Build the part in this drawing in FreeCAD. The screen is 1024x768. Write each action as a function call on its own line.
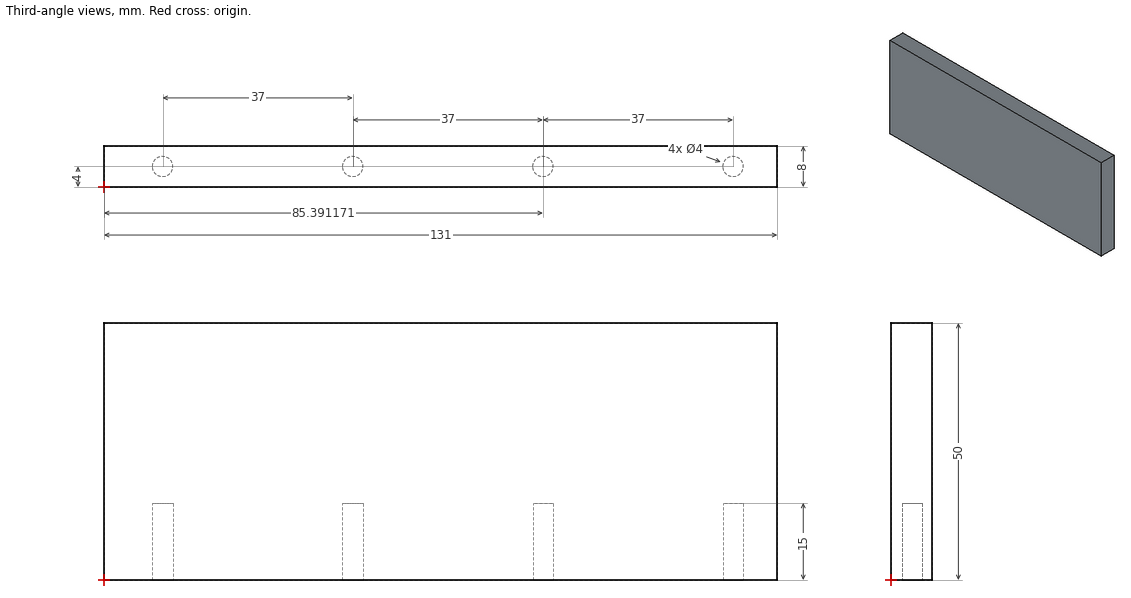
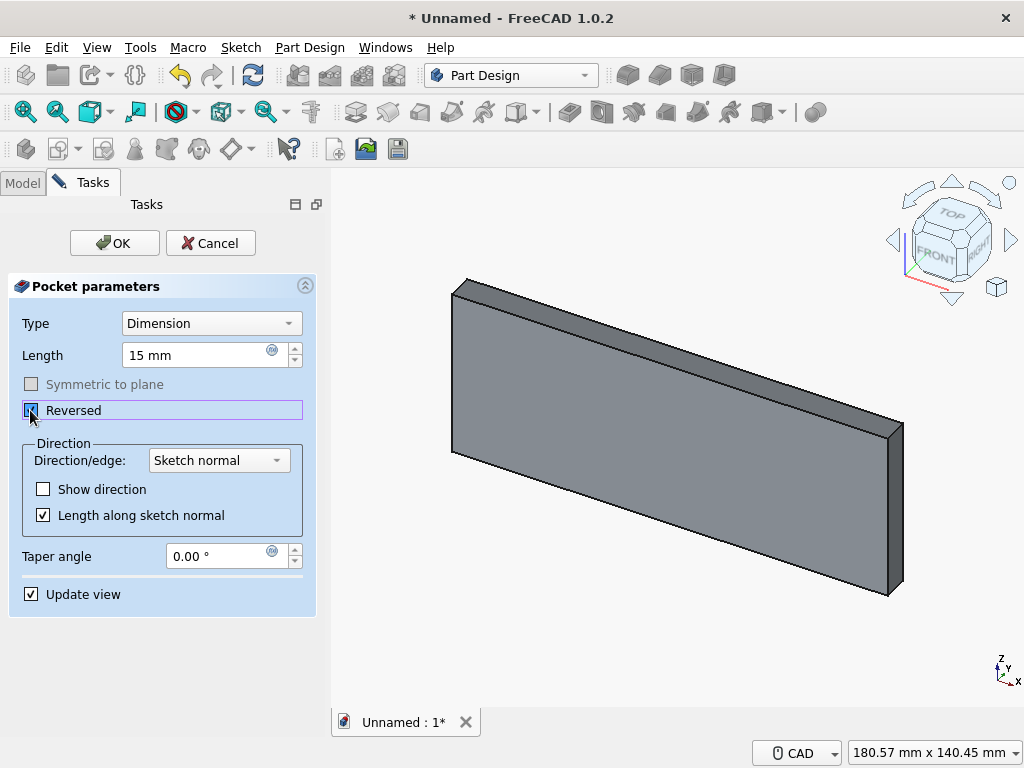
click(115, 243)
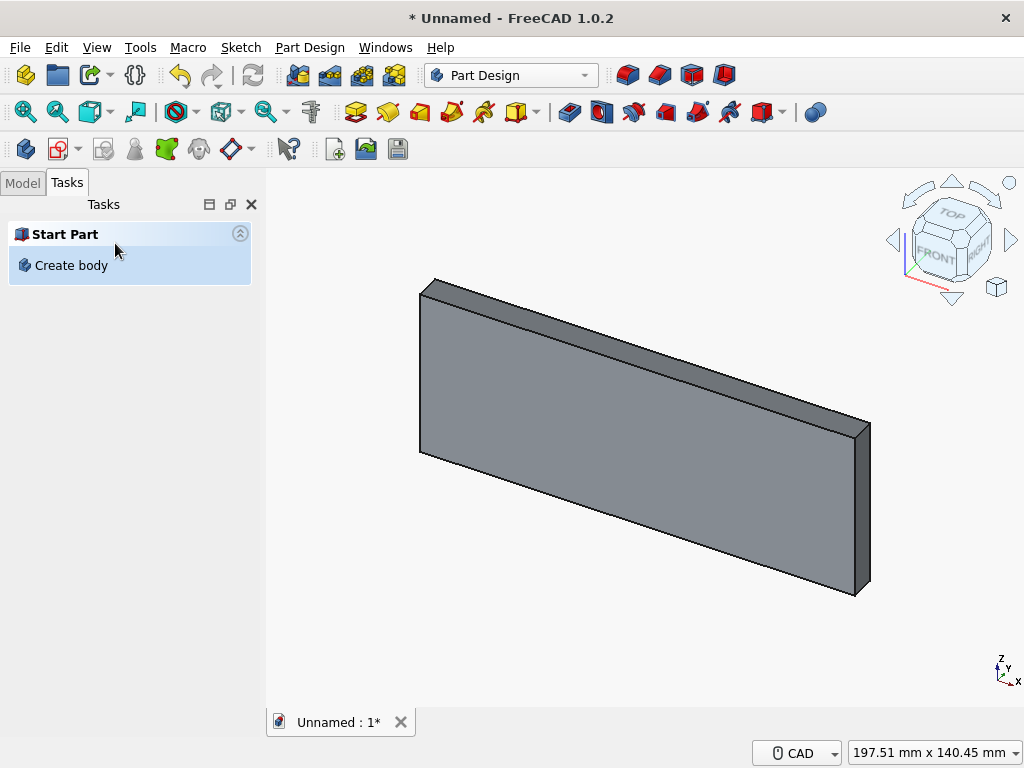
key(0)